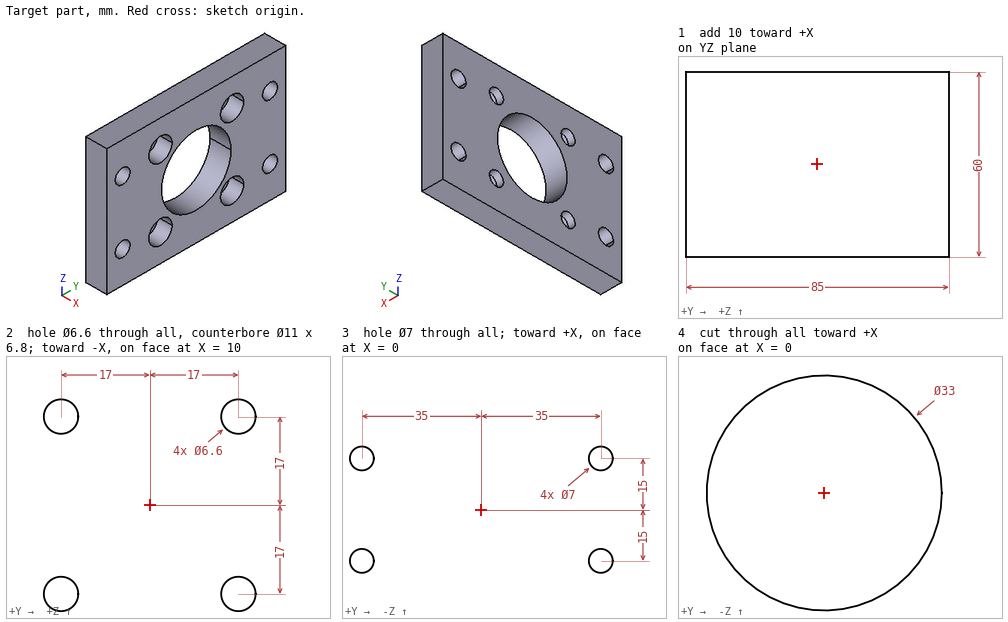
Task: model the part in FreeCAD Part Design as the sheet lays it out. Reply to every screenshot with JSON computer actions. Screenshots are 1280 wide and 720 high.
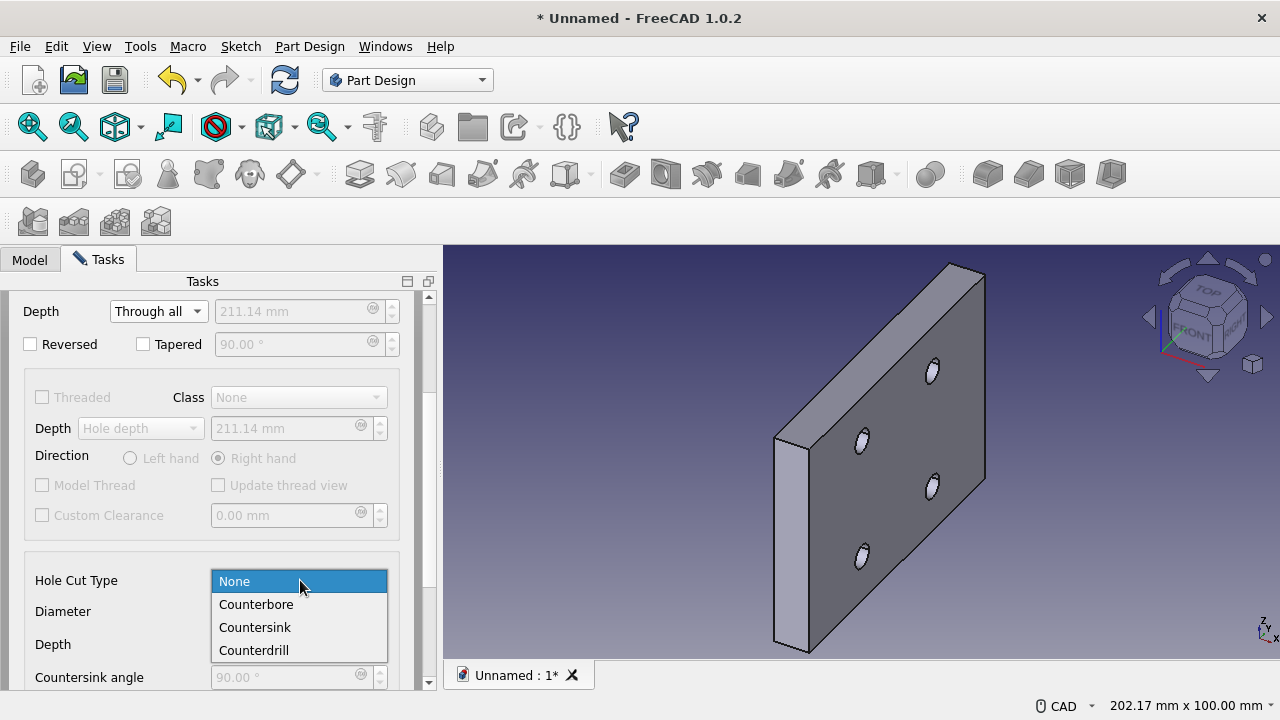
{"action": "left_click", "coordinate": [298, 604]}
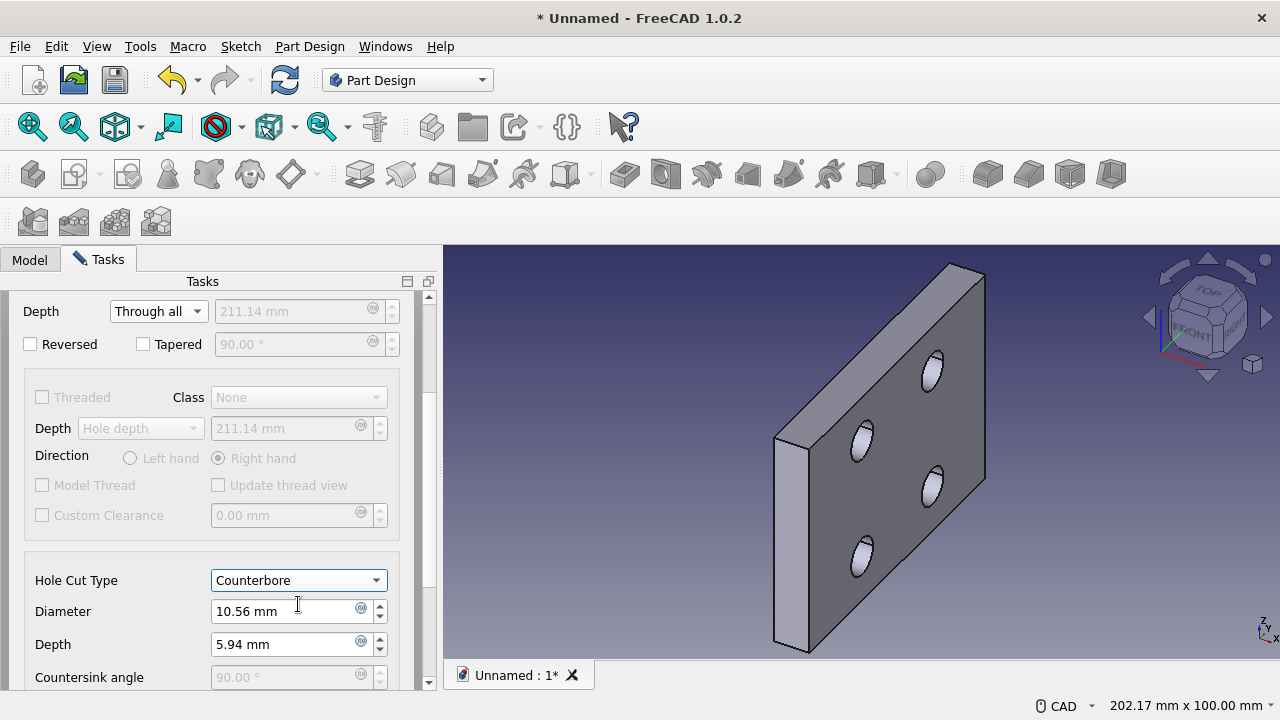
{"action": "triple_click", "coordinate": [292, 612]}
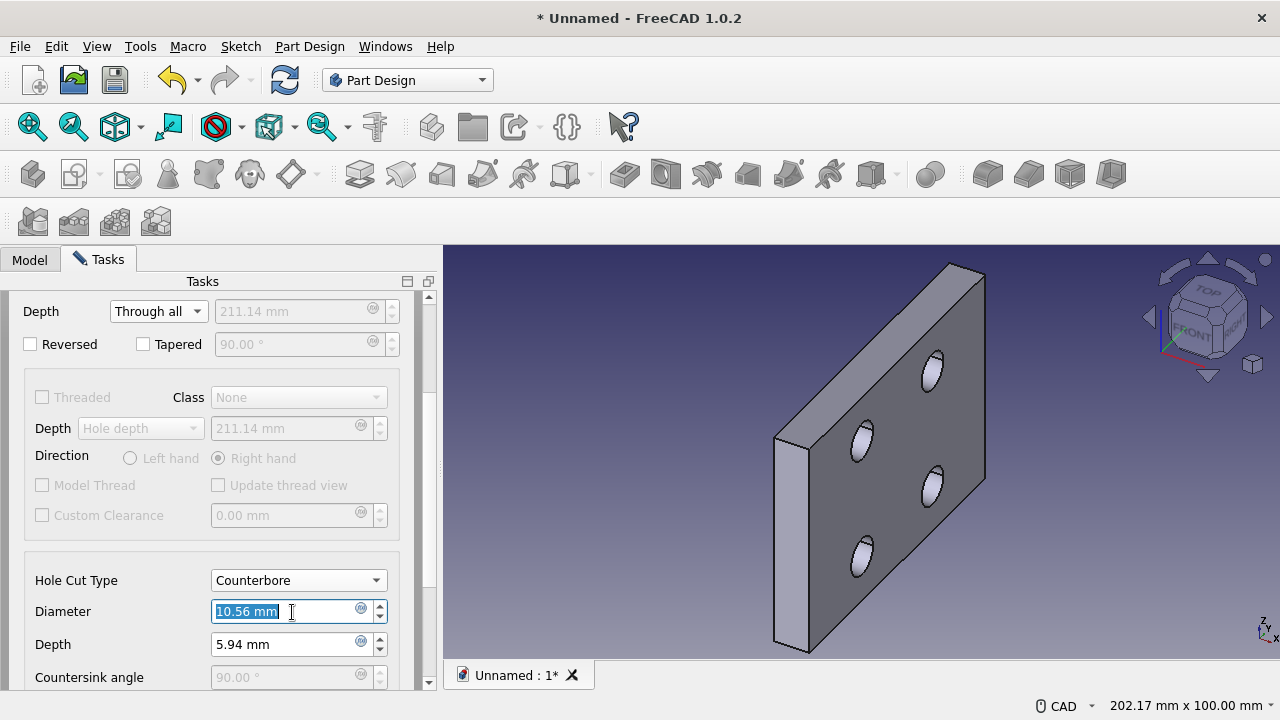
{"action": "type", "text": "11"}
{"action": "key", "text": "Tab"}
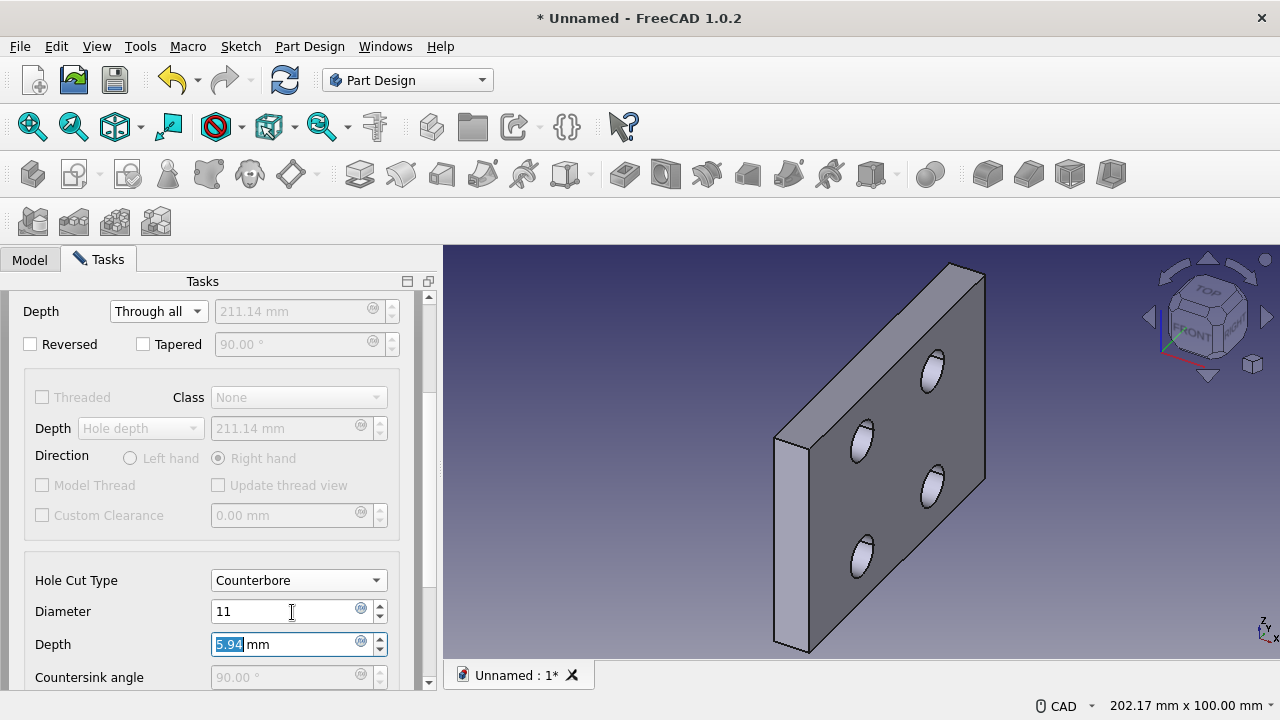
{"action": "type", "text": "6.8"}
{"action": "key", "text": "Tab"}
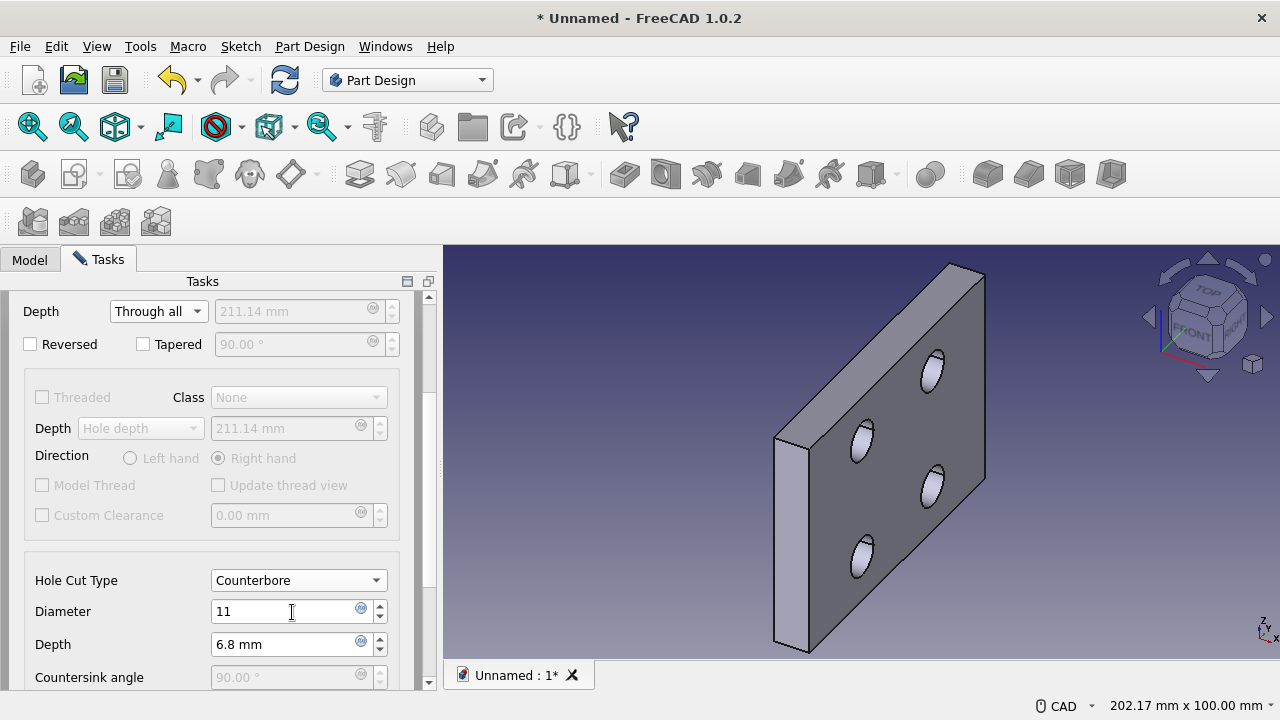
{"action": "scroll", "coordinate": [429, 490], "scroll_direction": "up", "scroll_amount": 4}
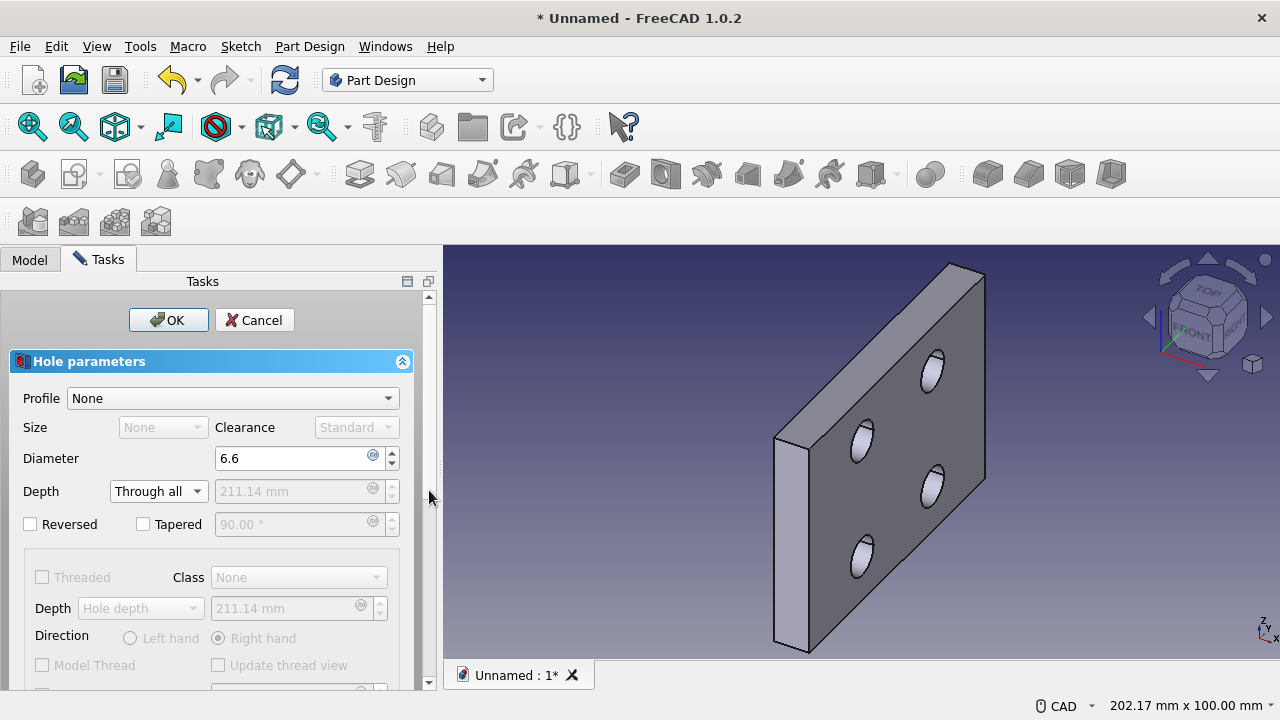
{"action": "left_click", "coordinate": [169, 320]}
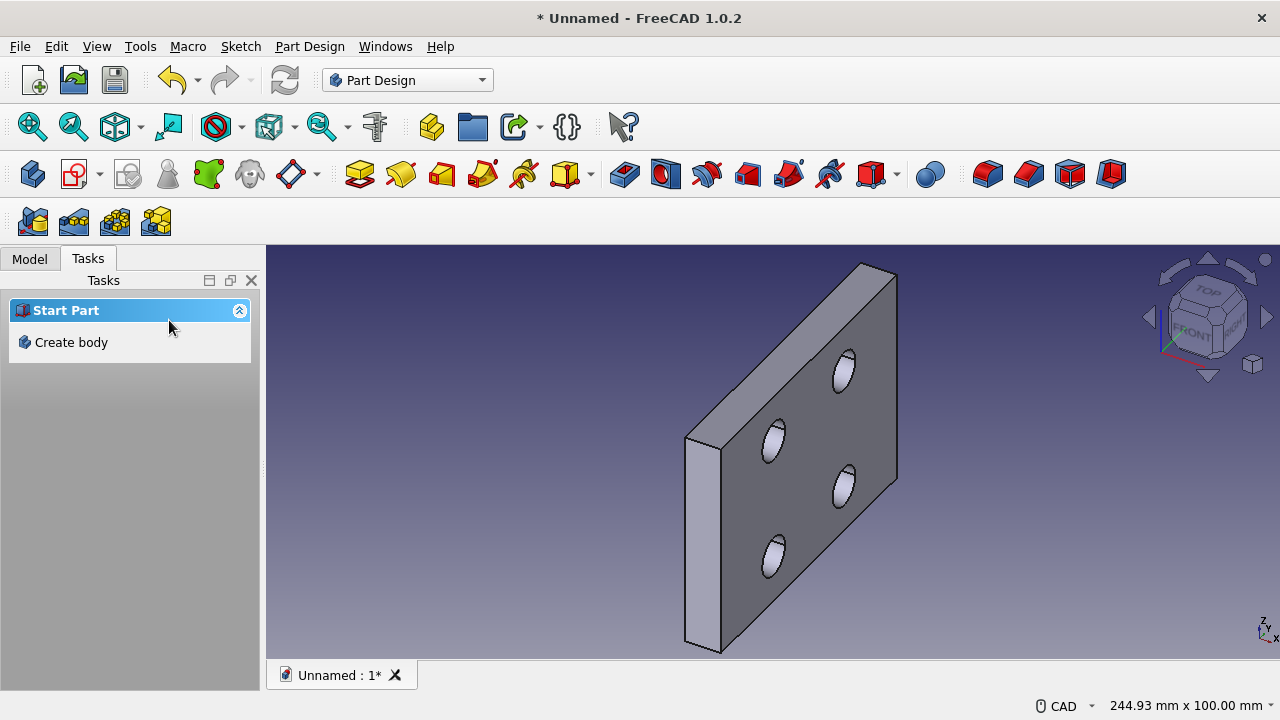
{"action": "key", "text": "6"}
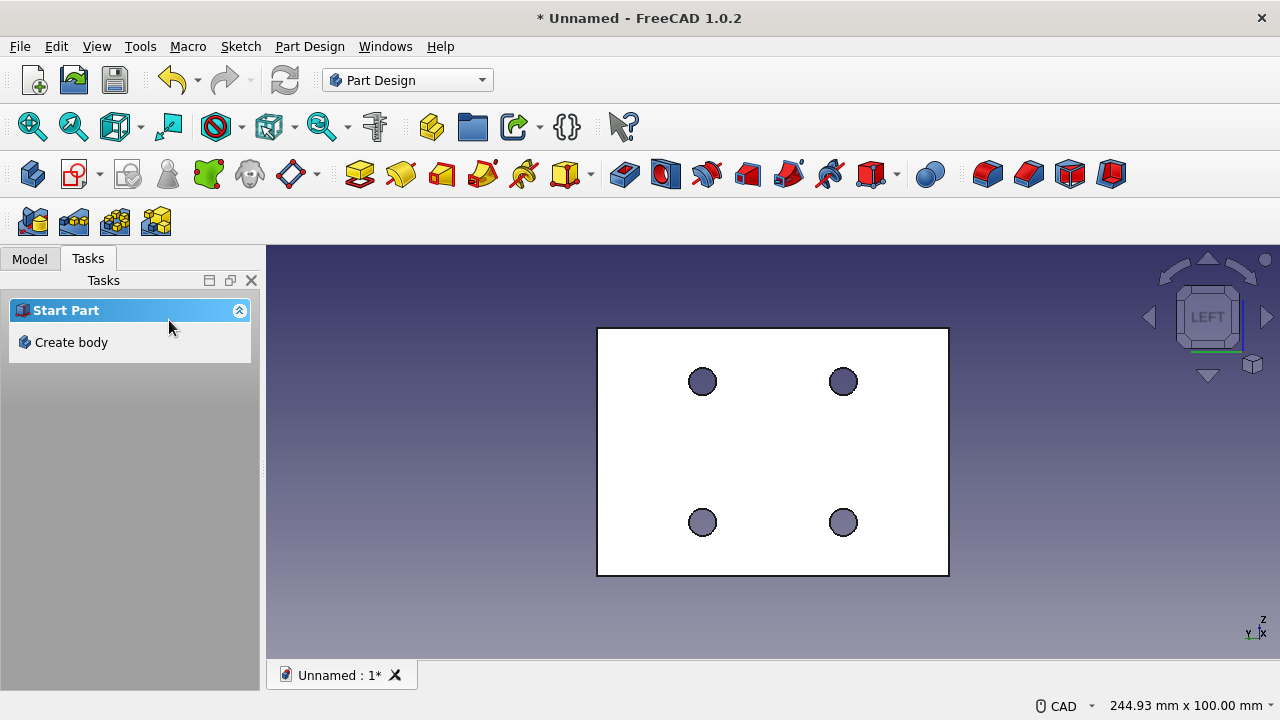
{"action": "left_click", "coordinate": [773, 451]}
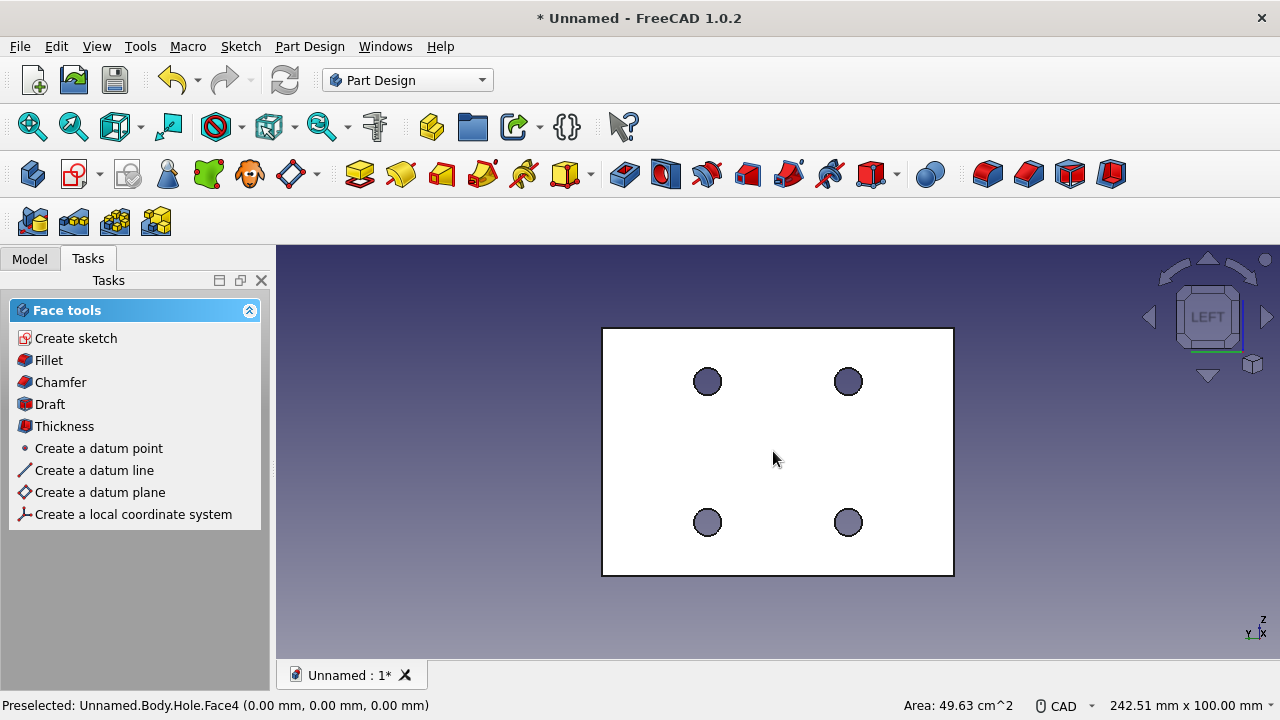
{"action": "left_click", "coordinate": [74, 174]}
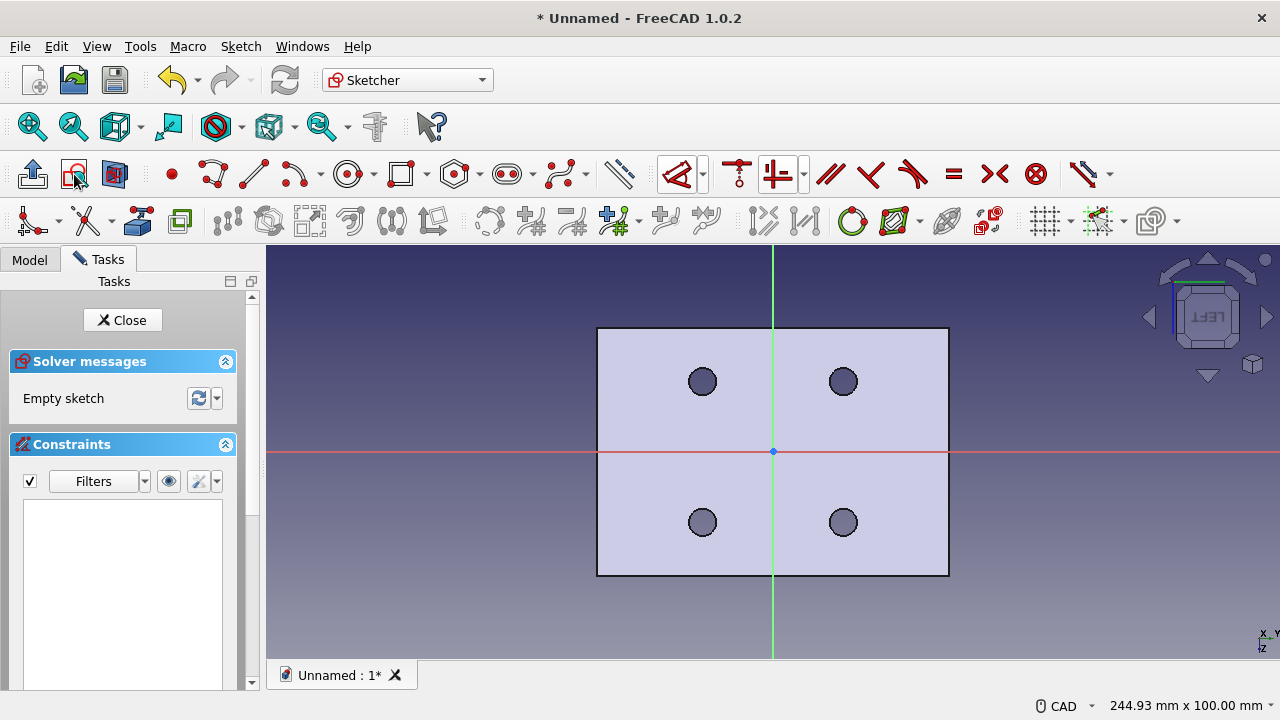
{"action": "scroll", "coordinate": [856, 452], "scroll_direction": "up", "scroll_amount": 3}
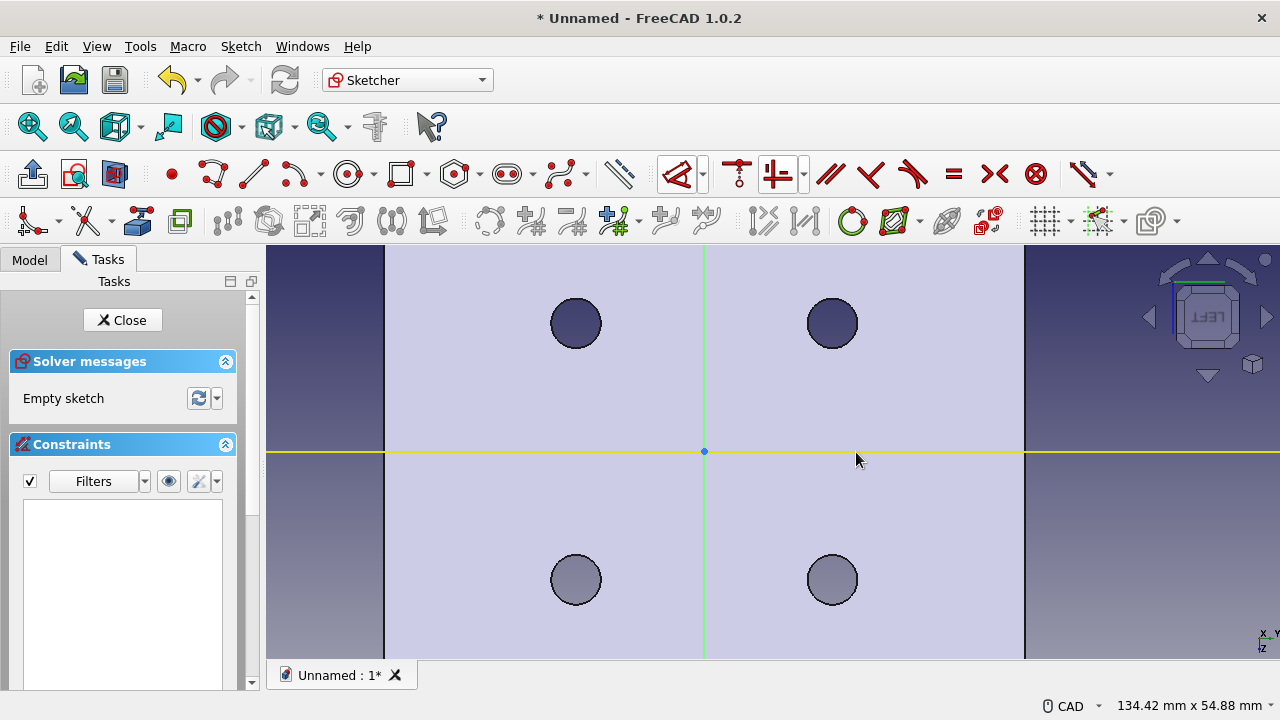
{"action": "left_click", "coordinate": [348, 174]}